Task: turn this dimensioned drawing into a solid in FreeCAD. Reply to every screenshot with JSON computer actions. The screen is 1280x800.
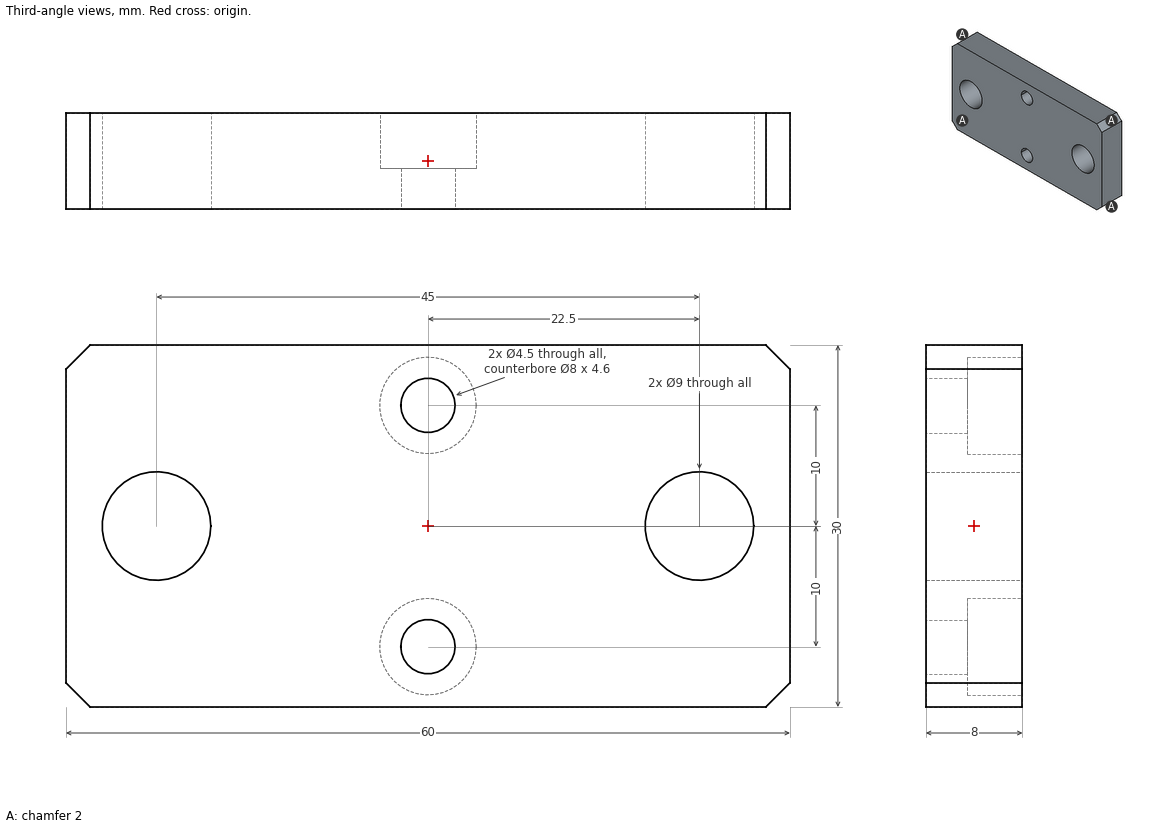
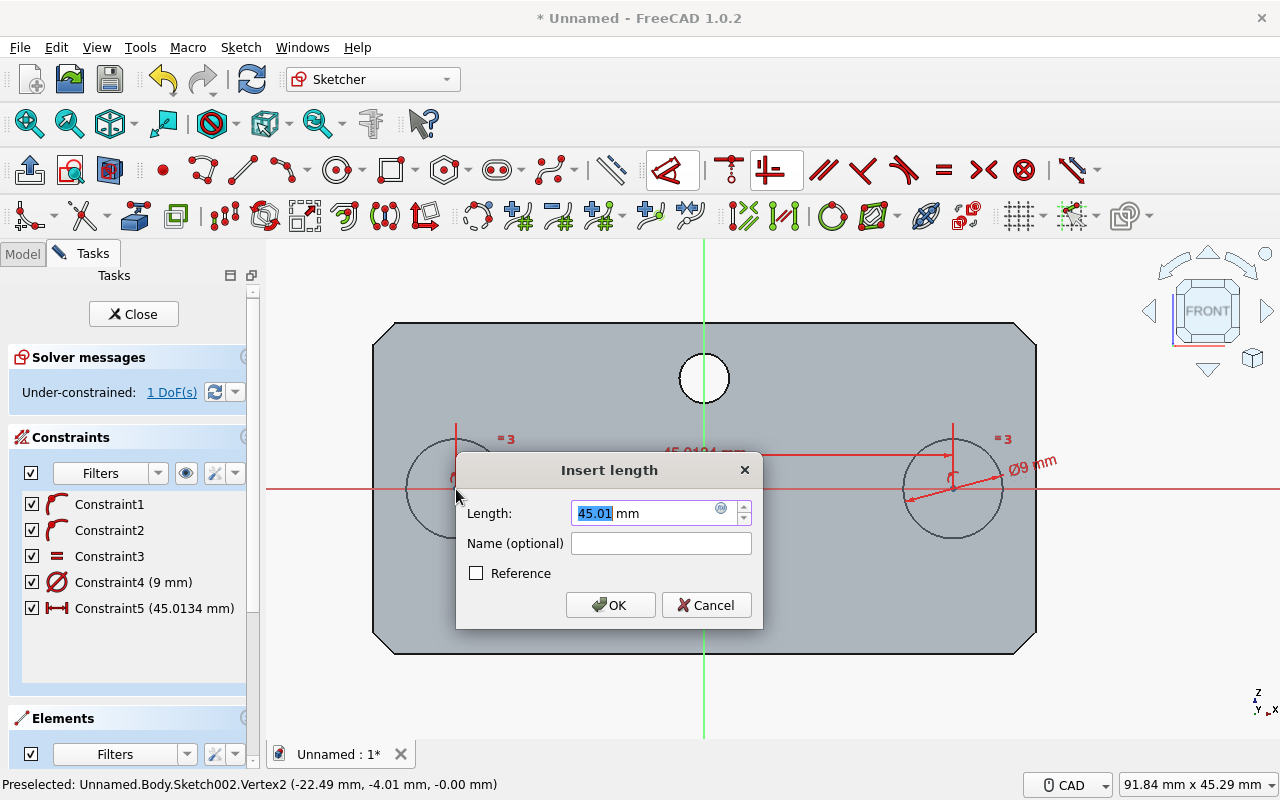
{"action": "type", "text": "45"}
{"action": "key", "text": "Return"}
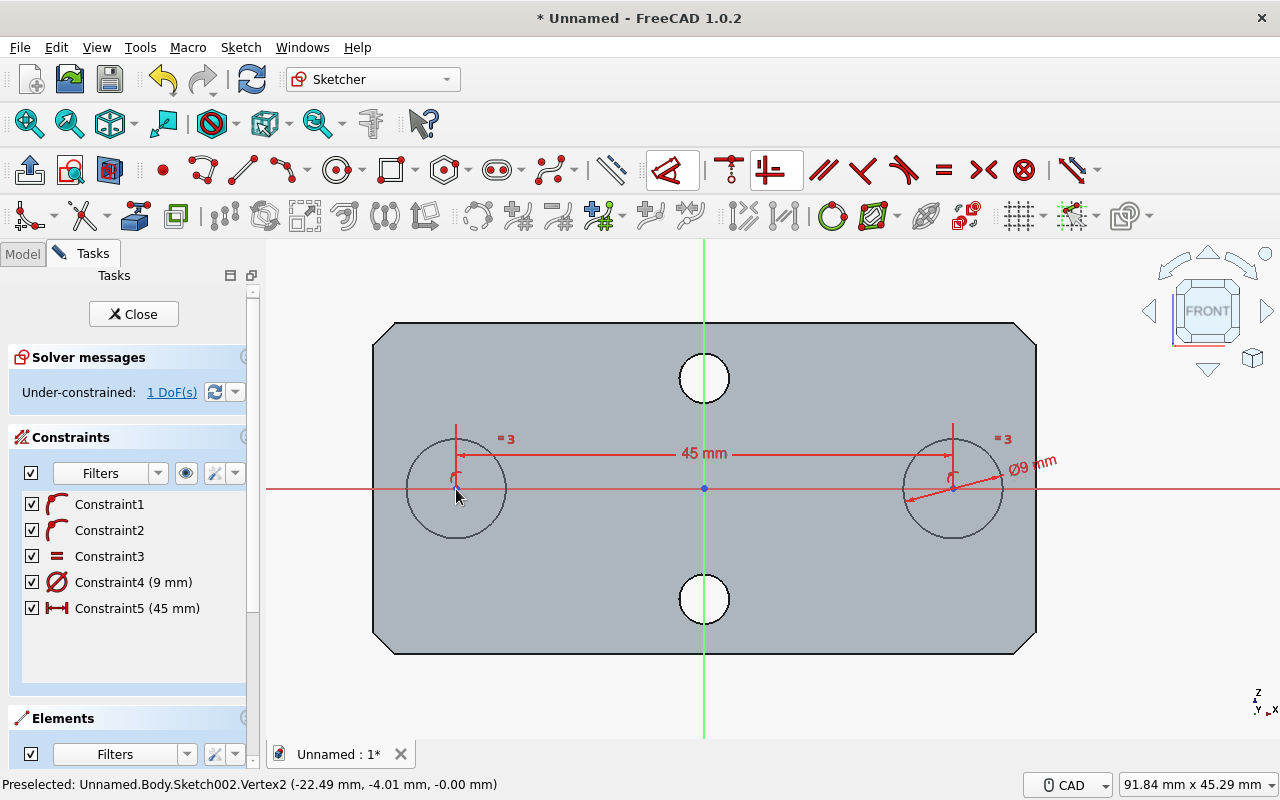
{"action": "left_click", "coordinate": [953, 489]}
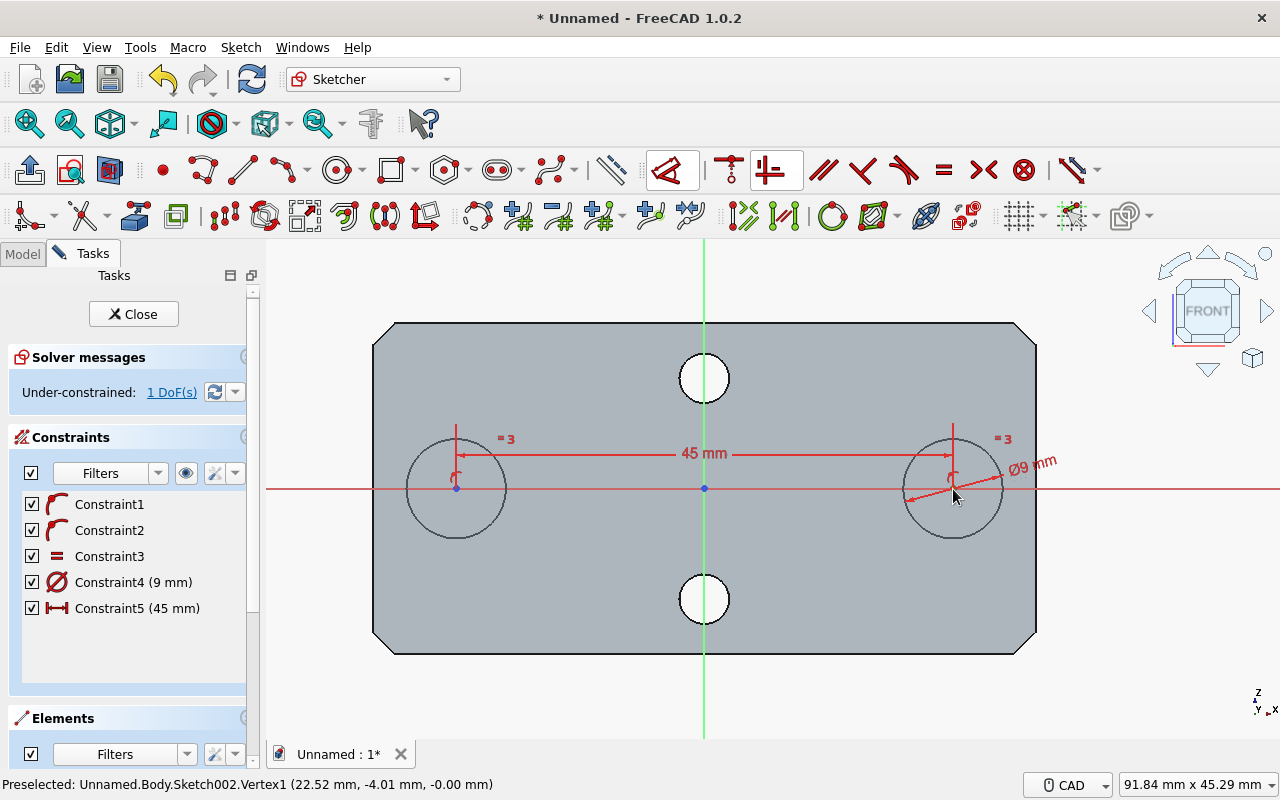
{"action": "left_click", "coordinate": [694, 170]}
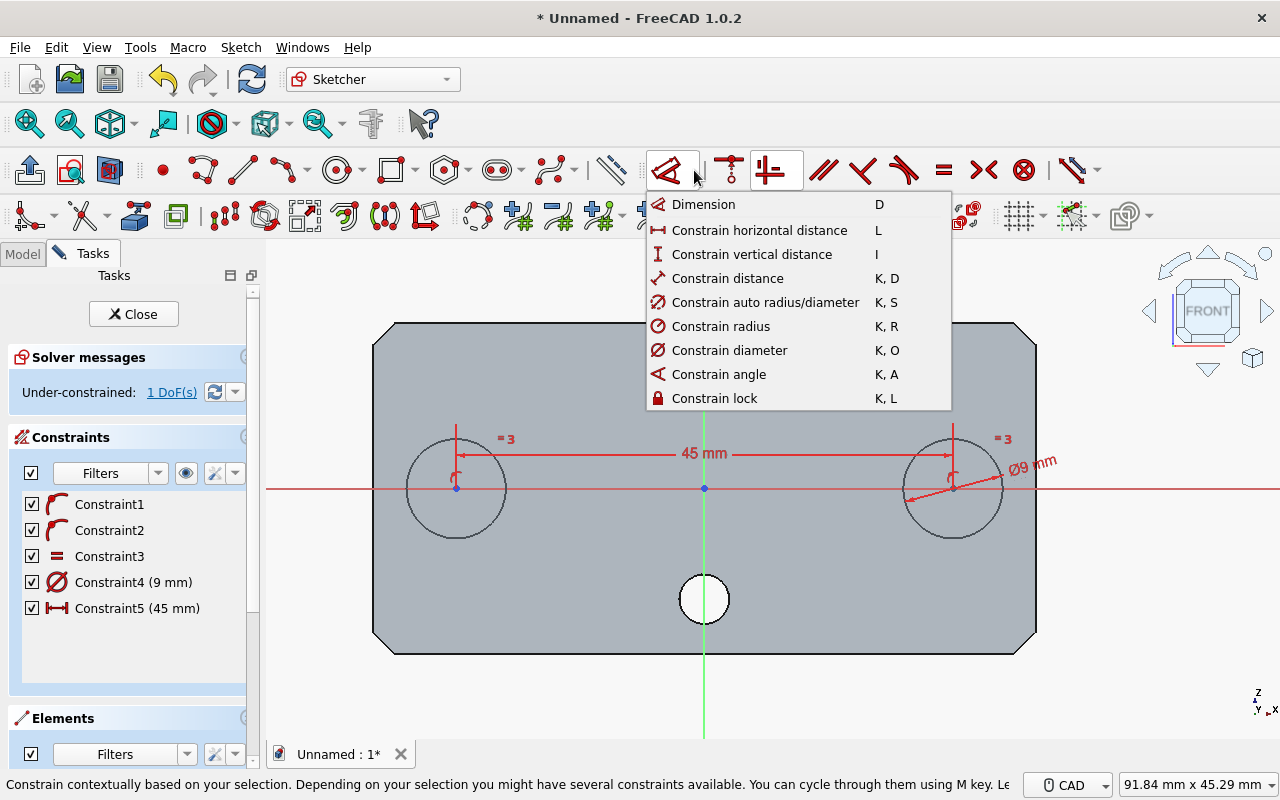
{"action": "left_click", "coordinate": [799, 230]}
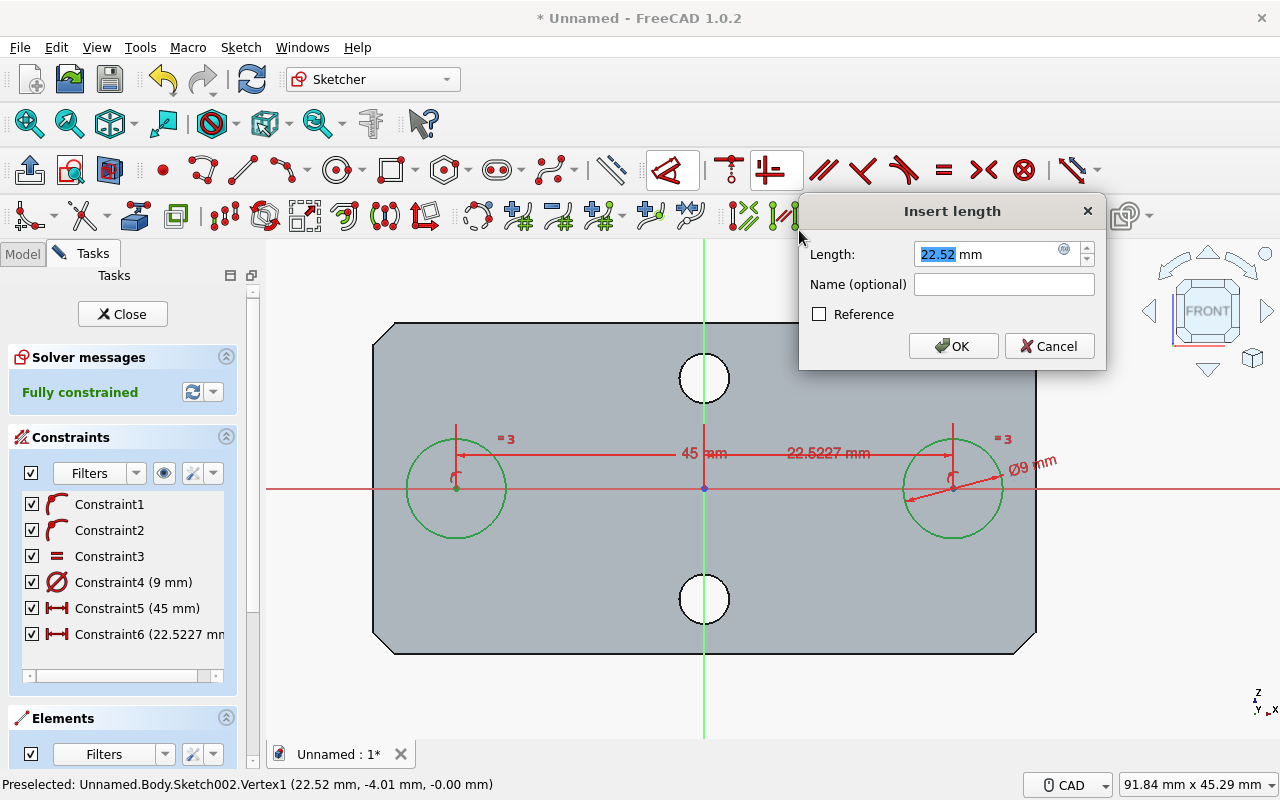
{"action": "type", "text": "22.5"}
{"action": "key", "text": "Return"}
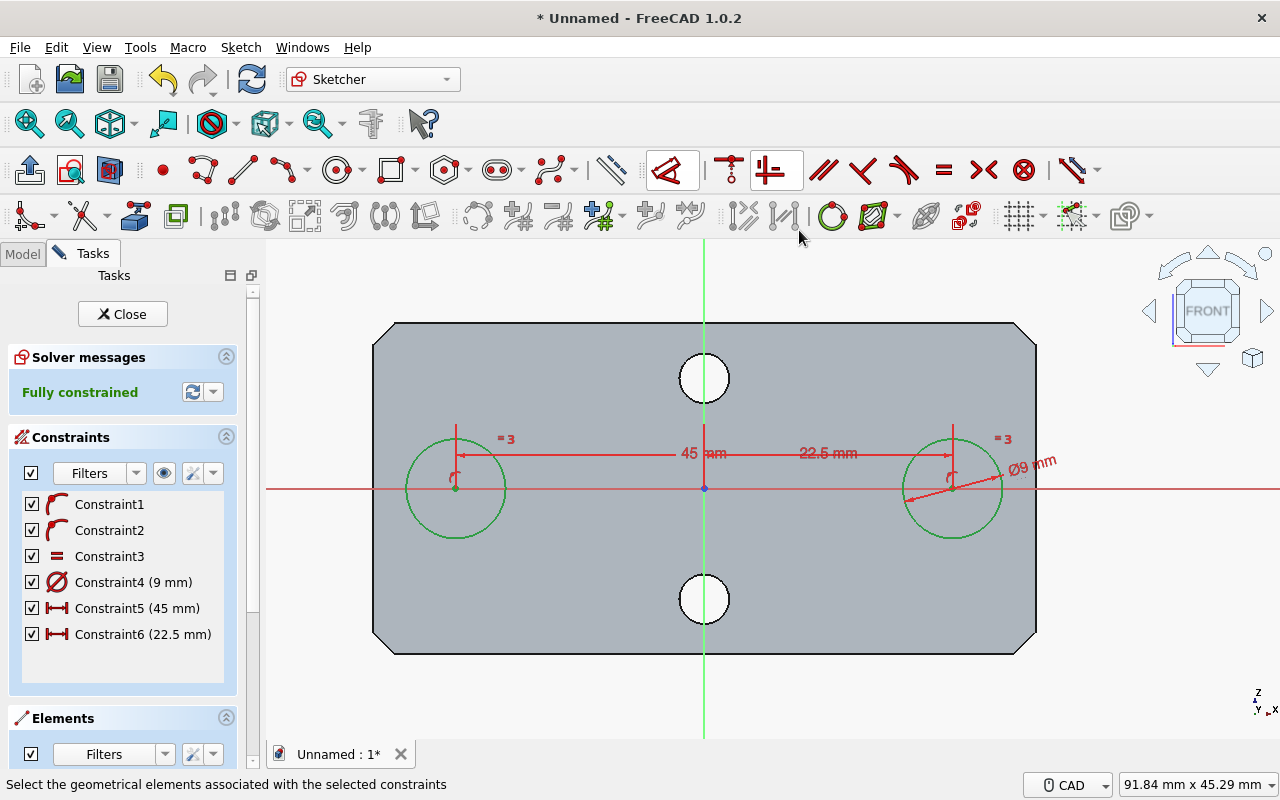
{"action": "left_click", "coordinate": [123, 314]}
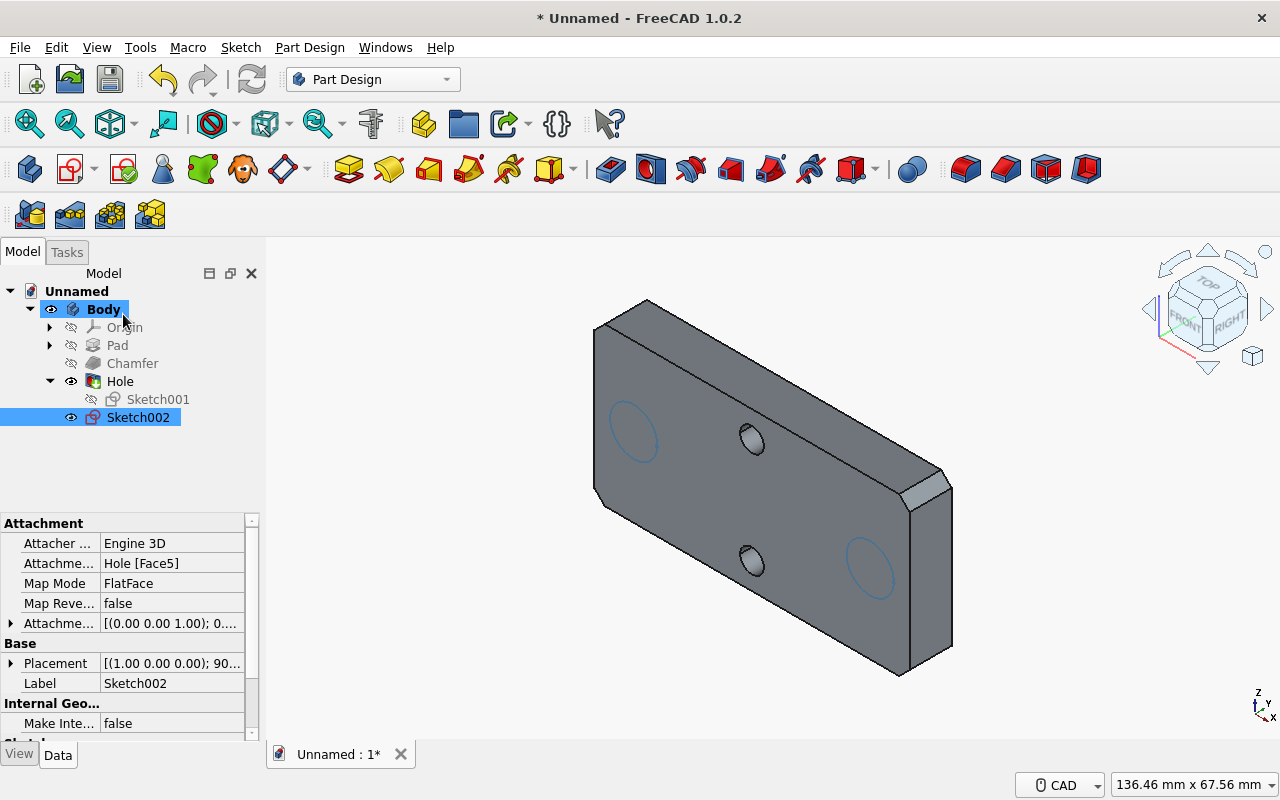
{"action": "left_click", "coordinate": [652, 170]}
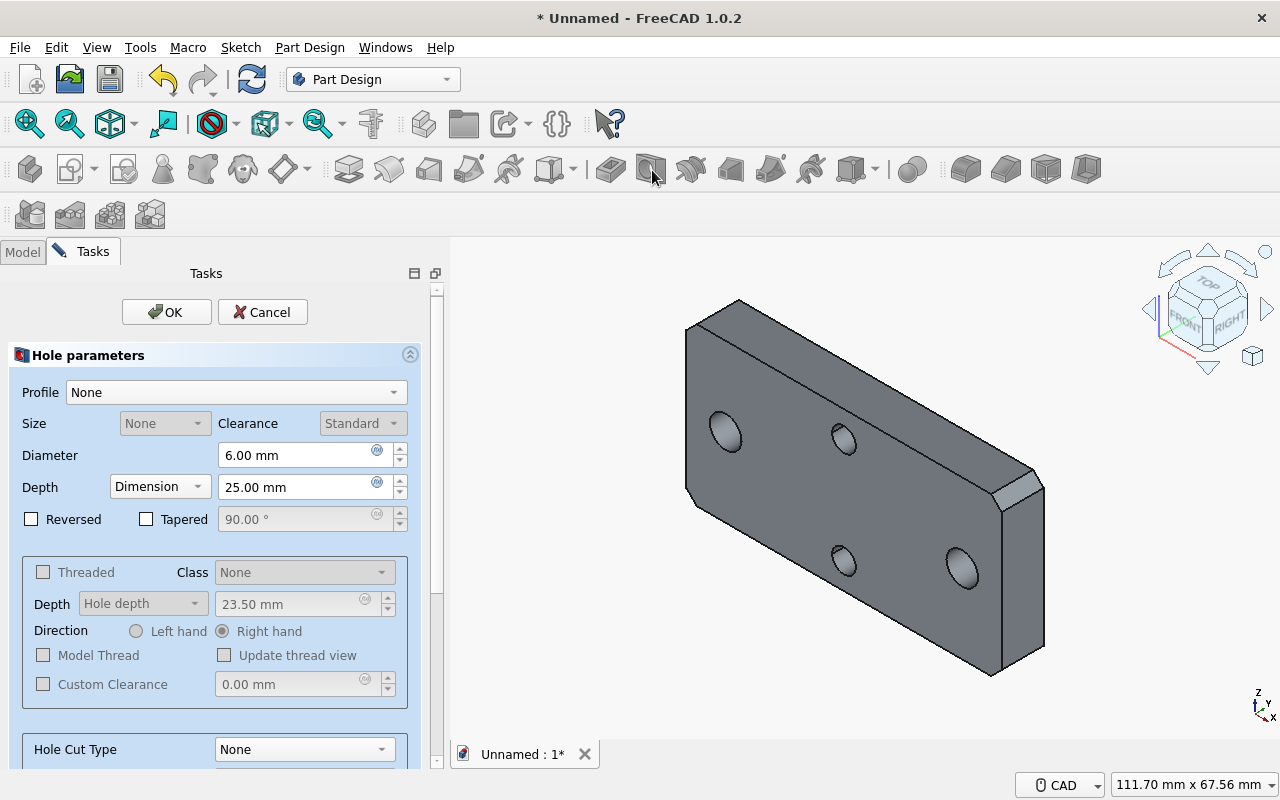
{"action": "triple_click", "coordinate": [305, 455]}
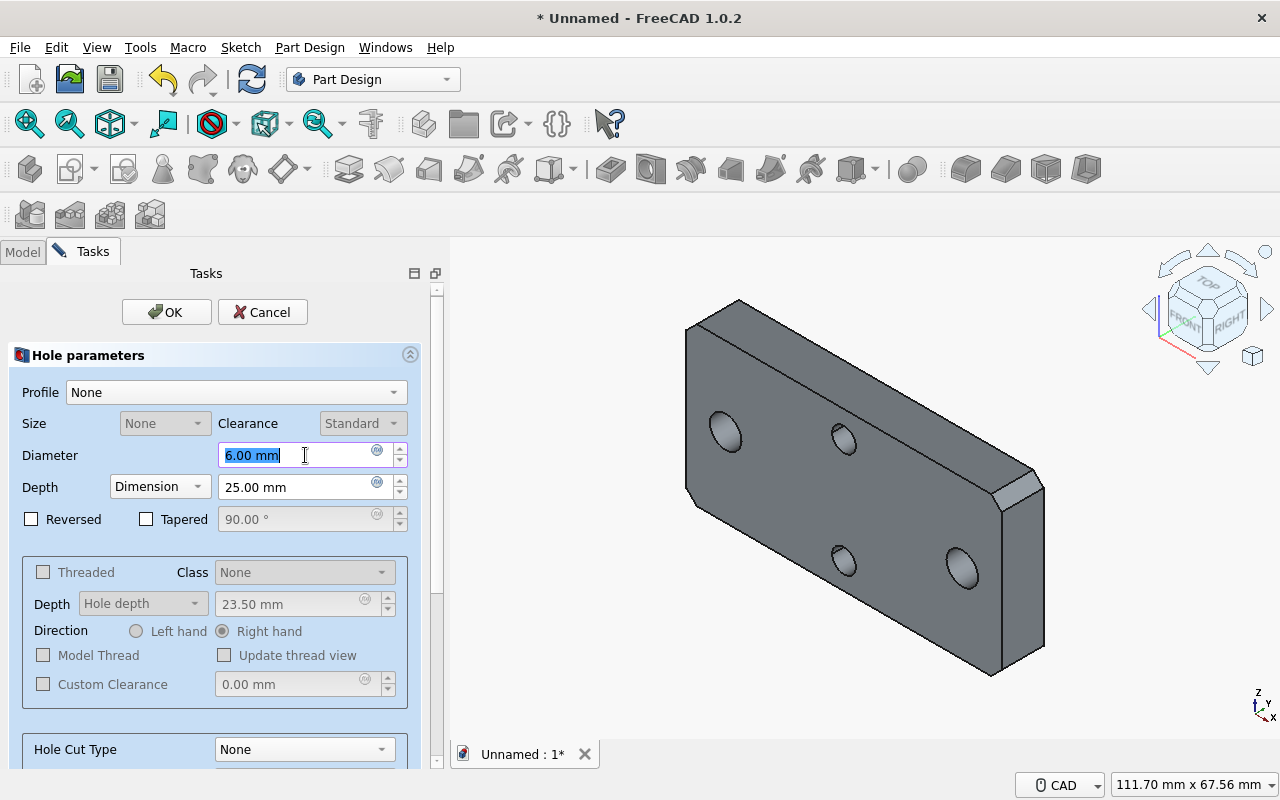
{"action": "type", "text": "9"}
{"action": "key", "text": "Tab"}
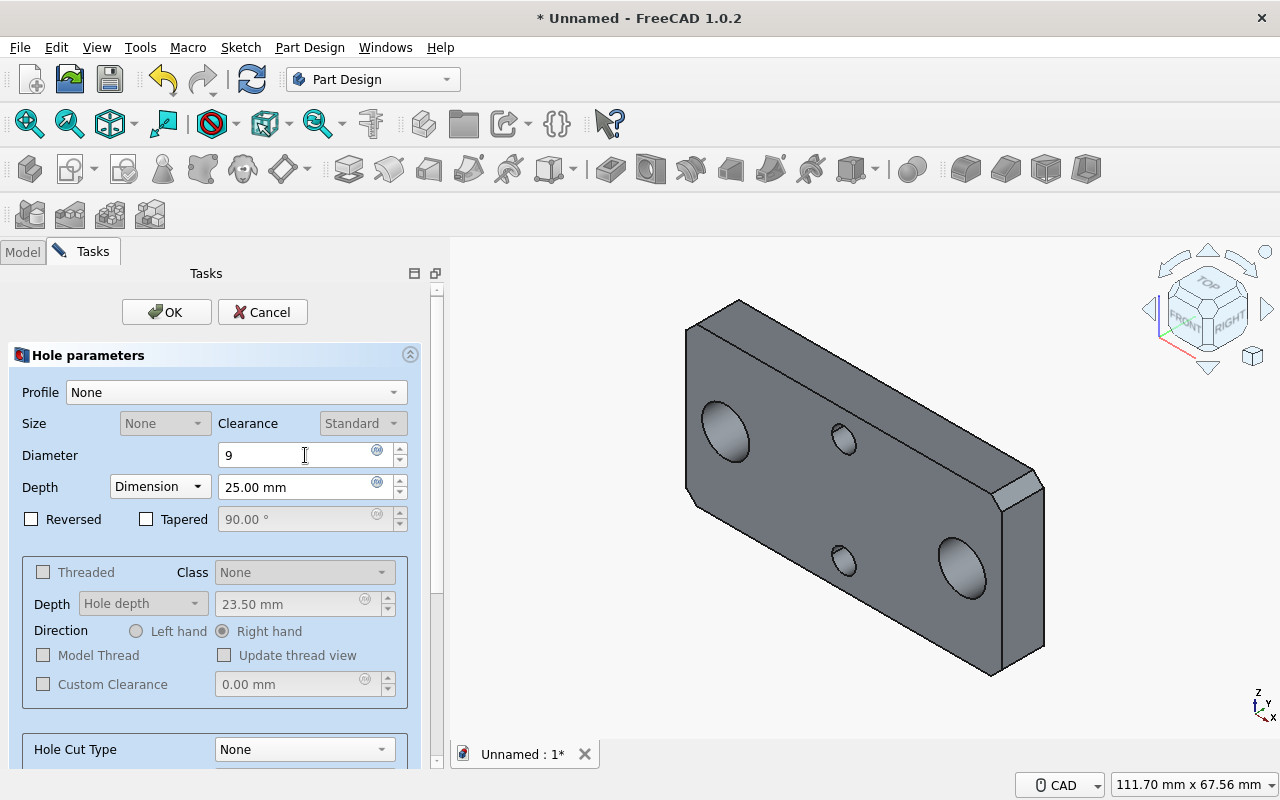
{"action": "left_click", "coordinate": [161, 486]}